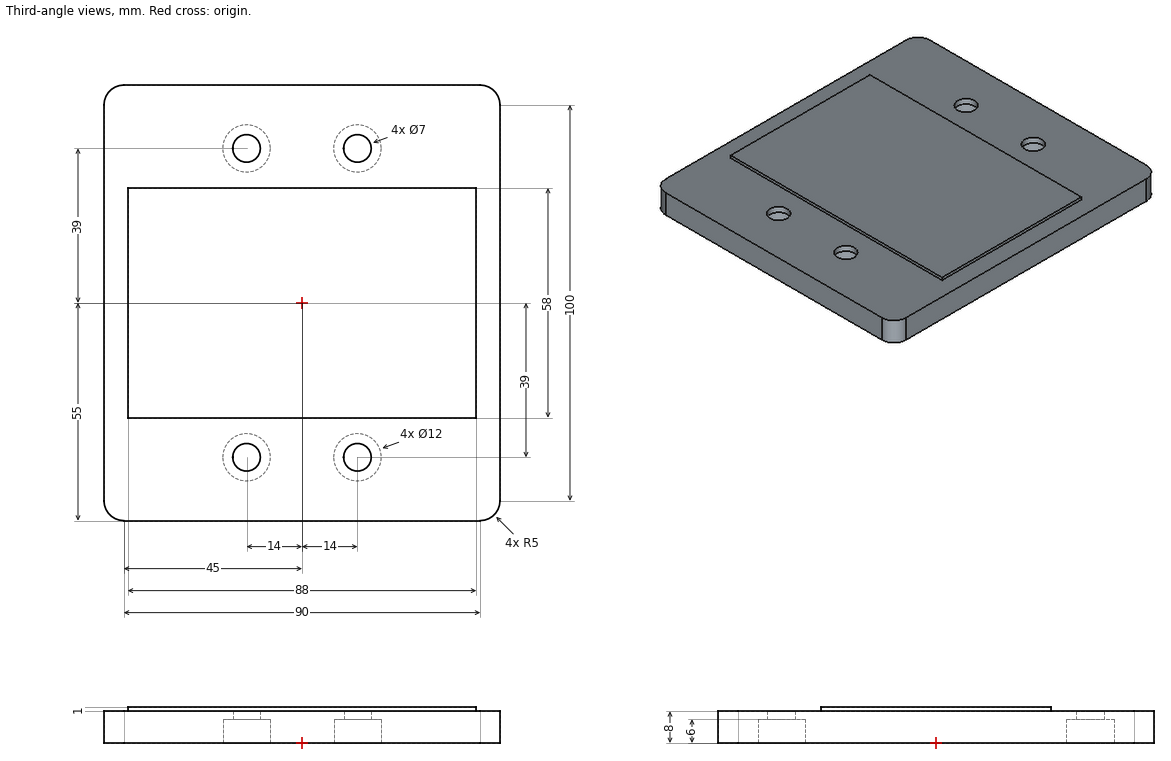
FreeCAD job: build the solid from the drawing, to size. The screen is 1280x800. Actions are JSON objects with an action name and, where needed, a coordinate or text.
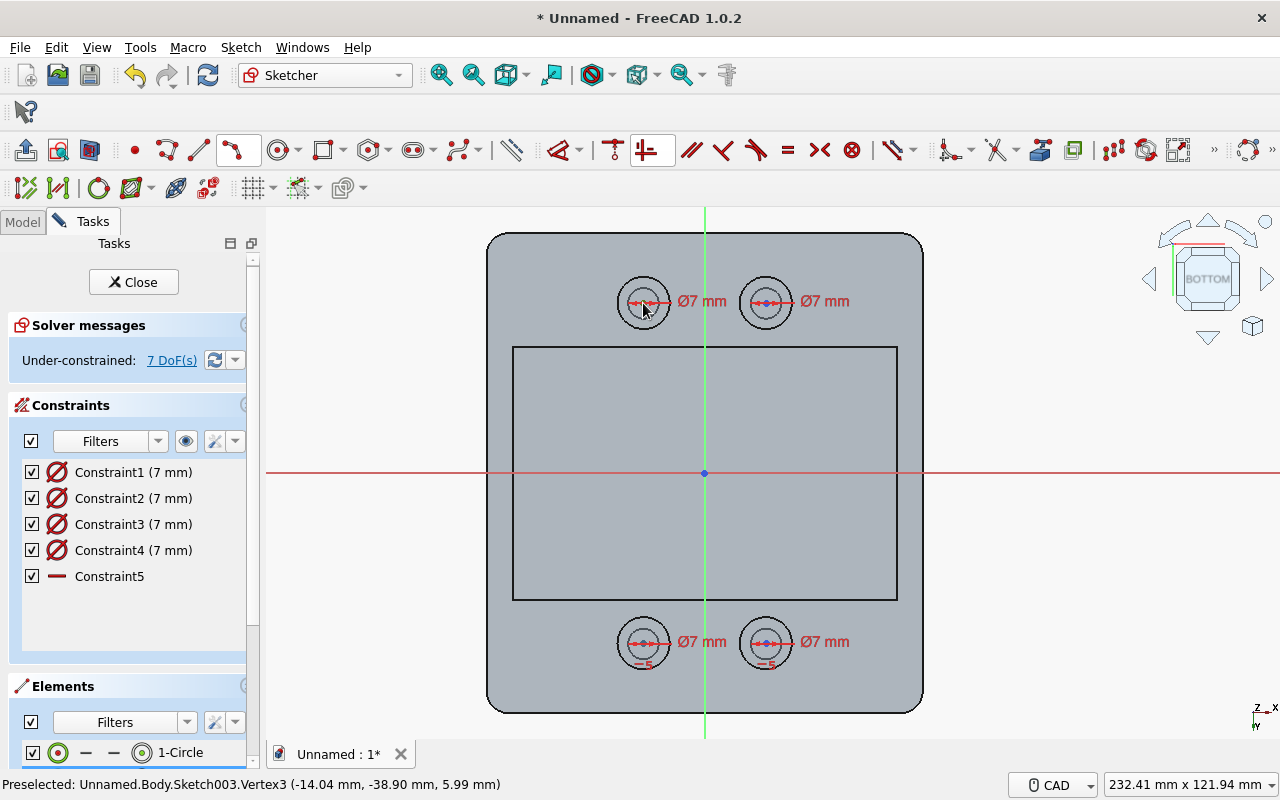
{"action": "key", "text": "v"}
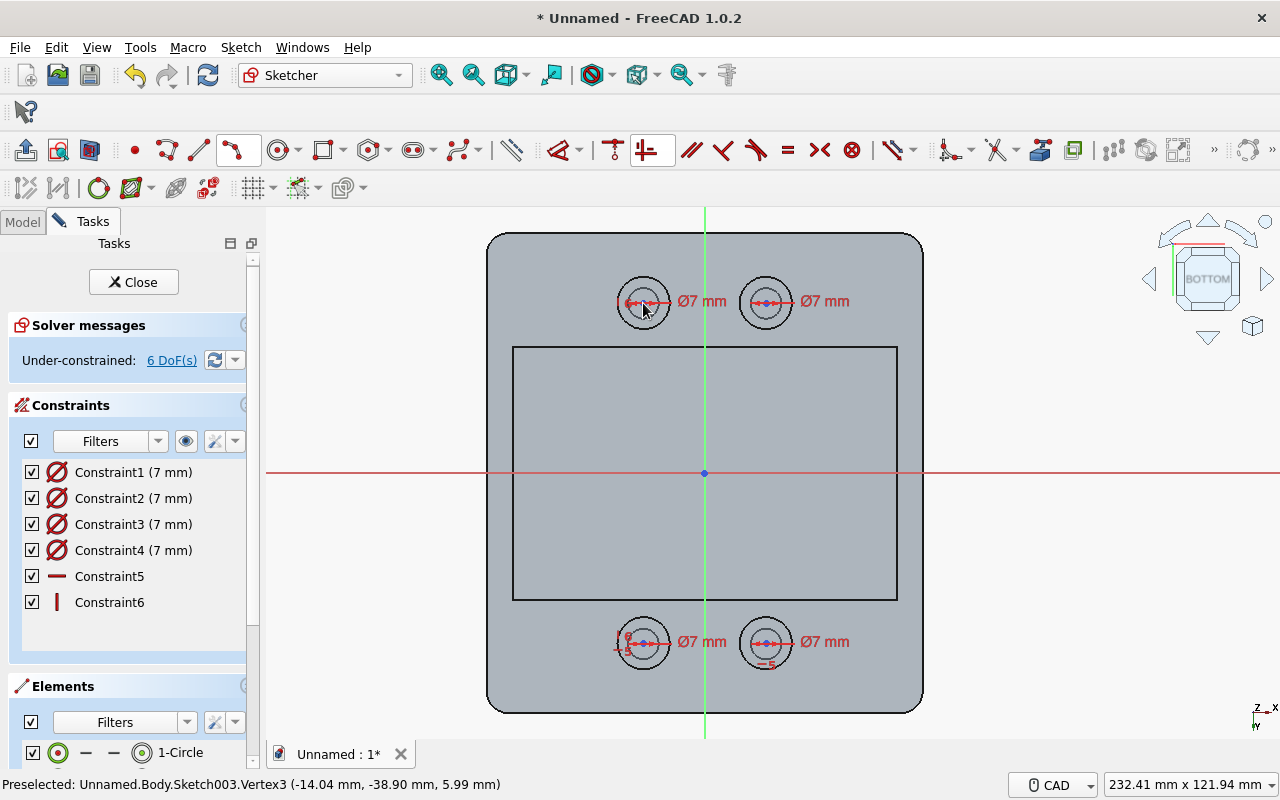
{"action": "left_click", "coordinate": [766, 644]}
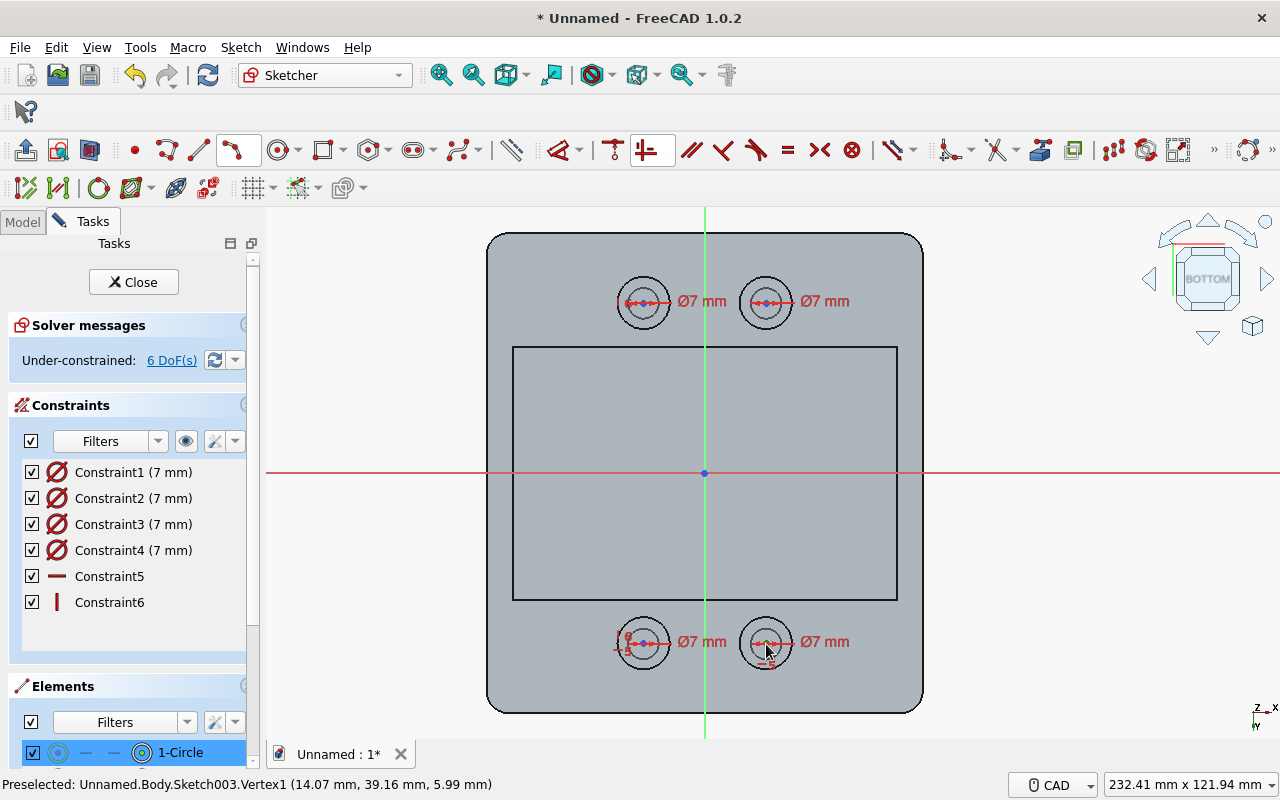
{"action": "left_click", "coordinate": [766, 303]}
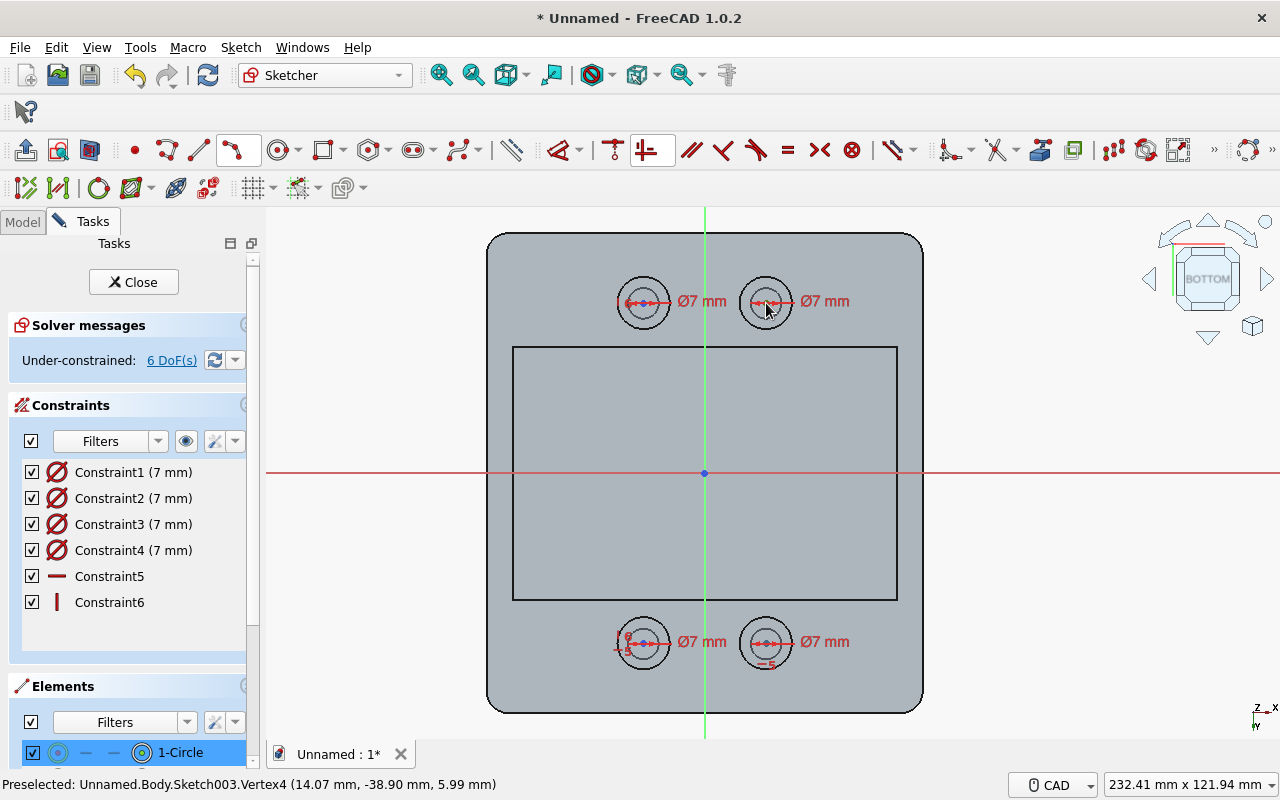
{"action": "key", "text": "v"}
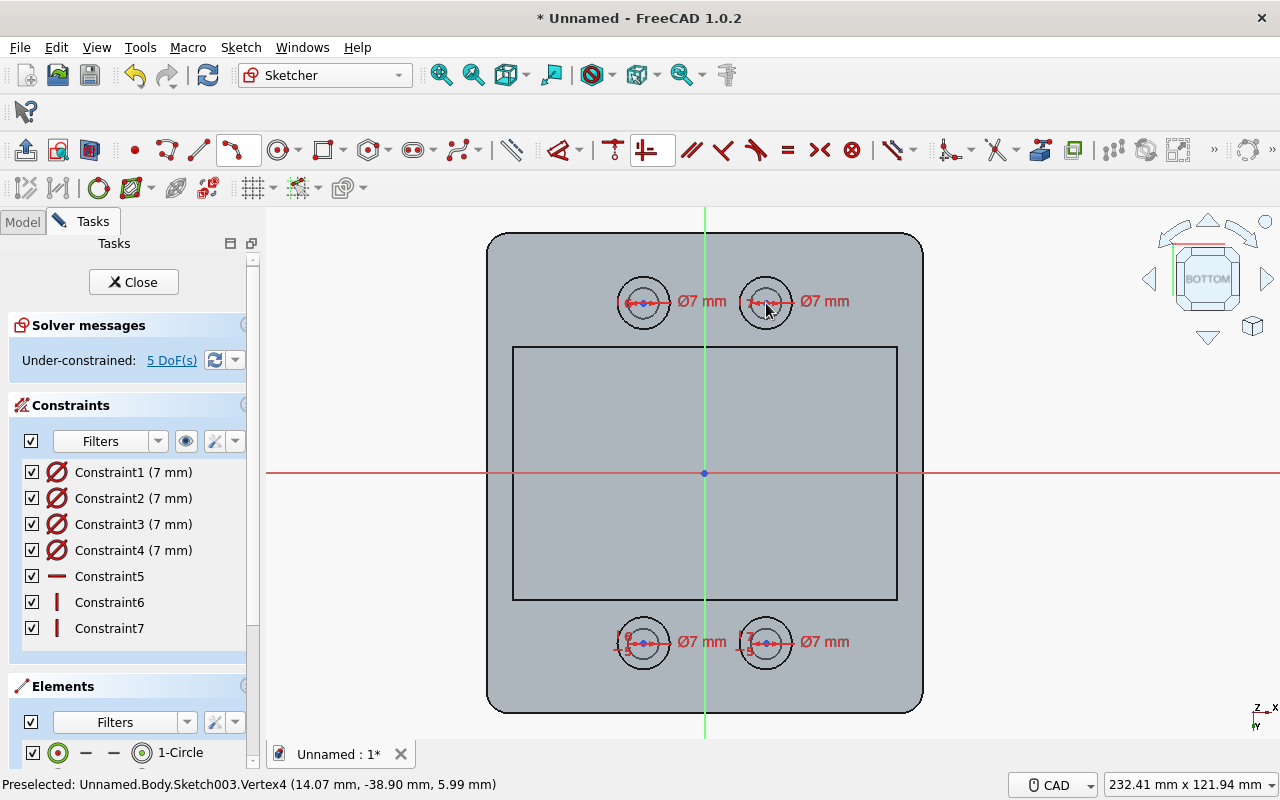
{"action": "left_click", "coordinate": [643, 303]}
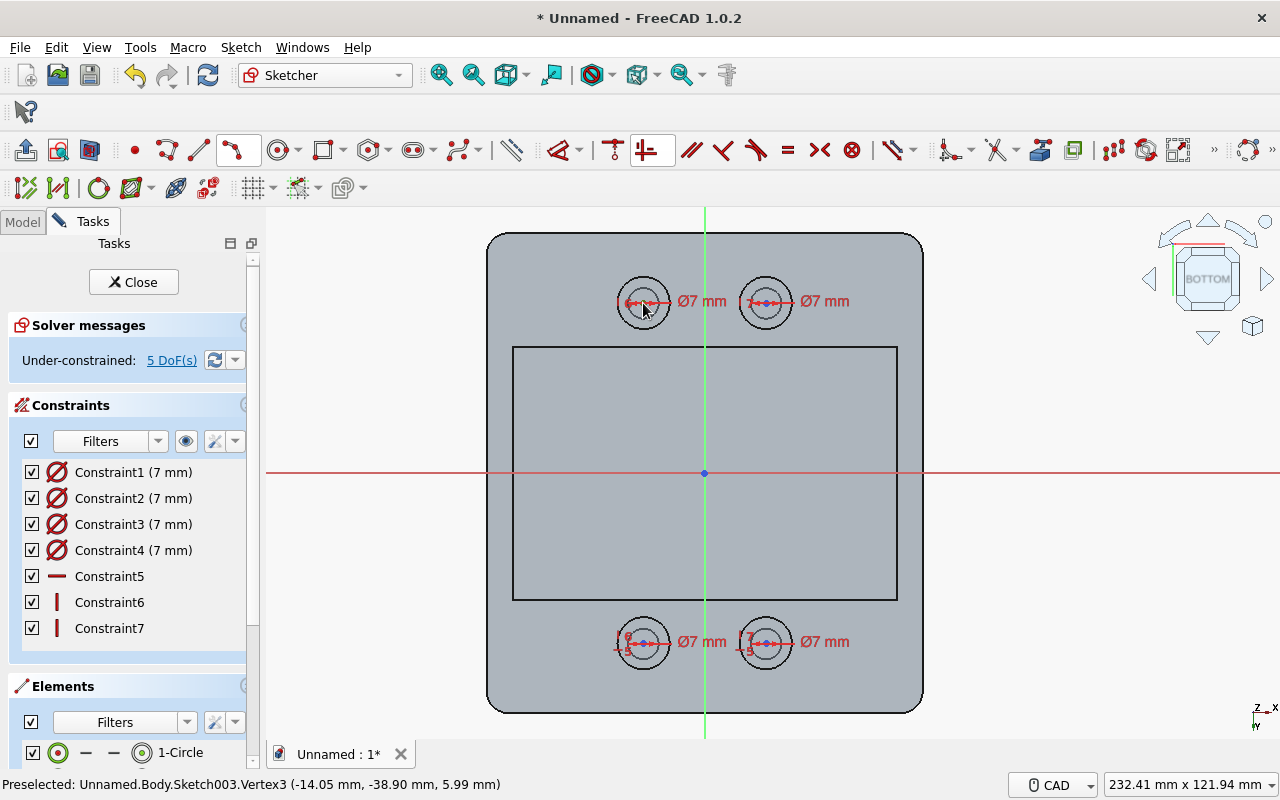
{"action": "left_click", "coordinate": [766, 303]}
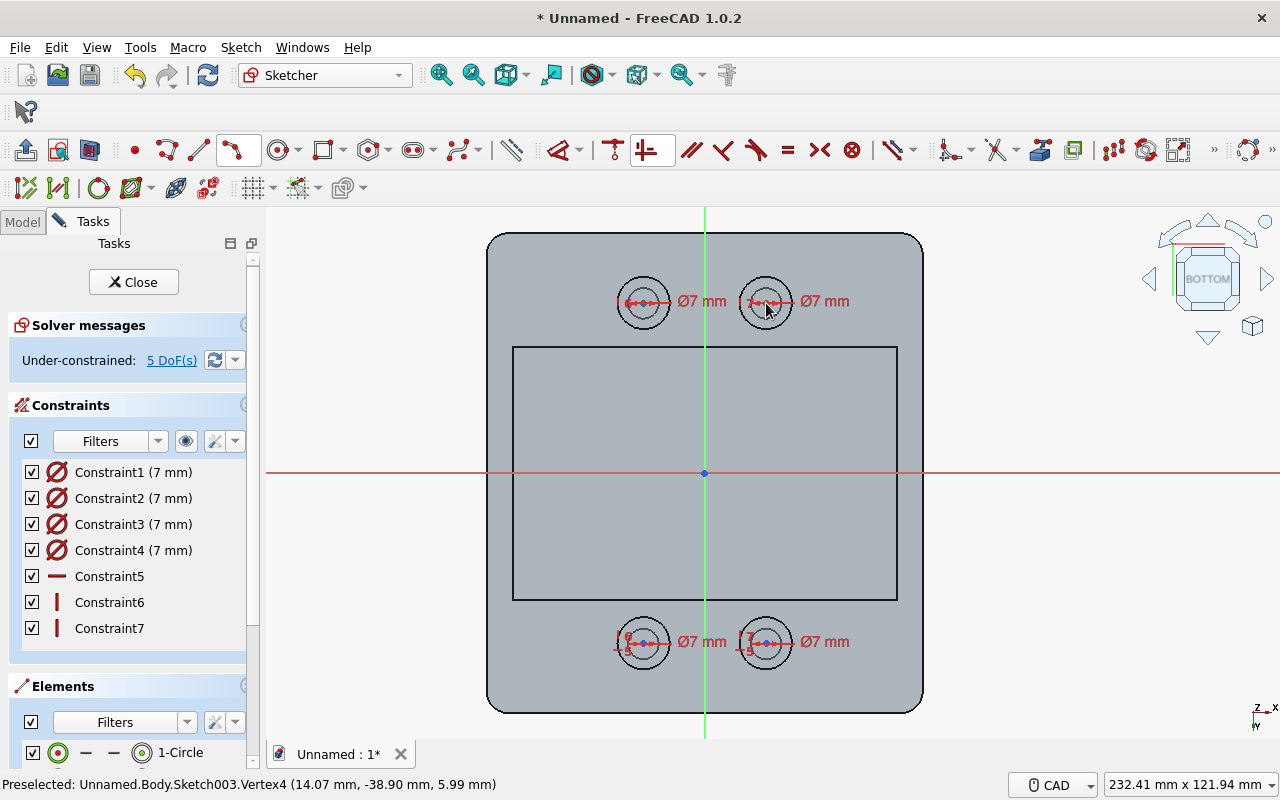
{"action": "key", "text": "h"}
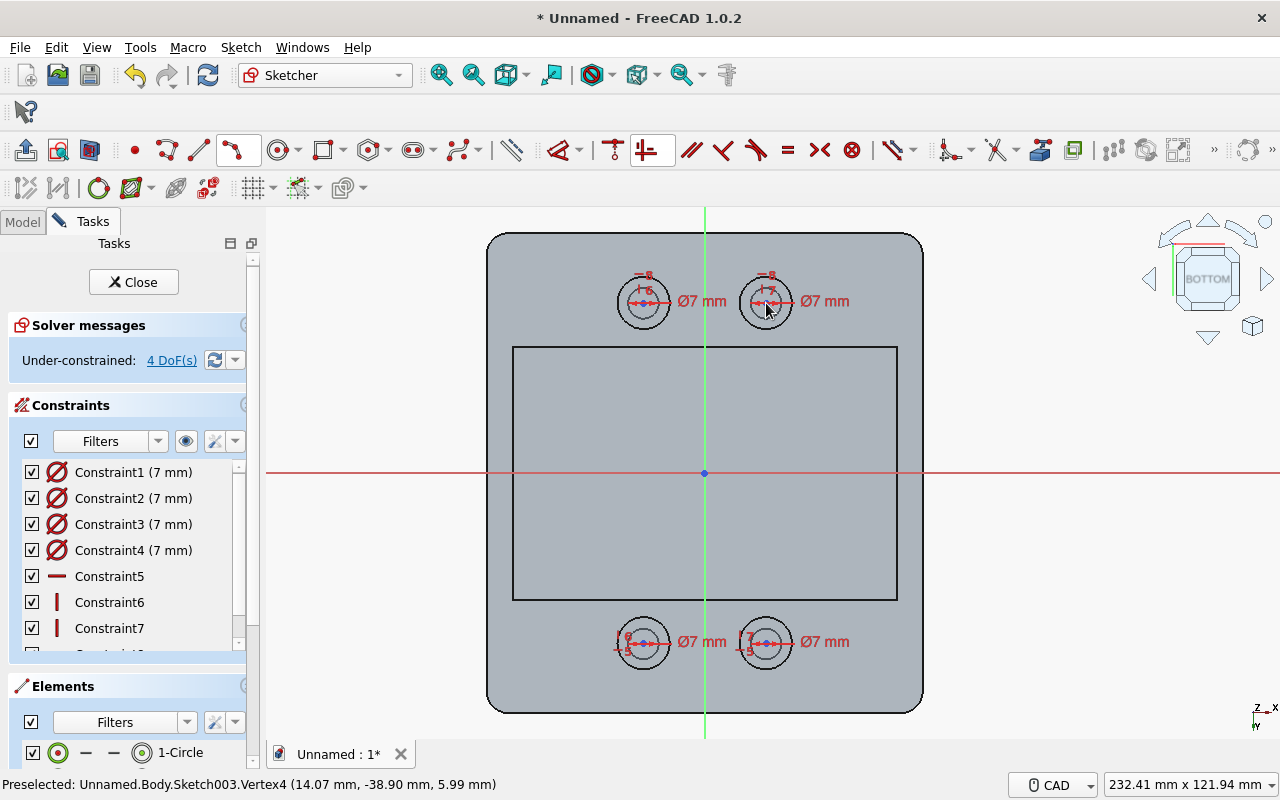
{"action": "left_click", "coordinate": [558, 150]}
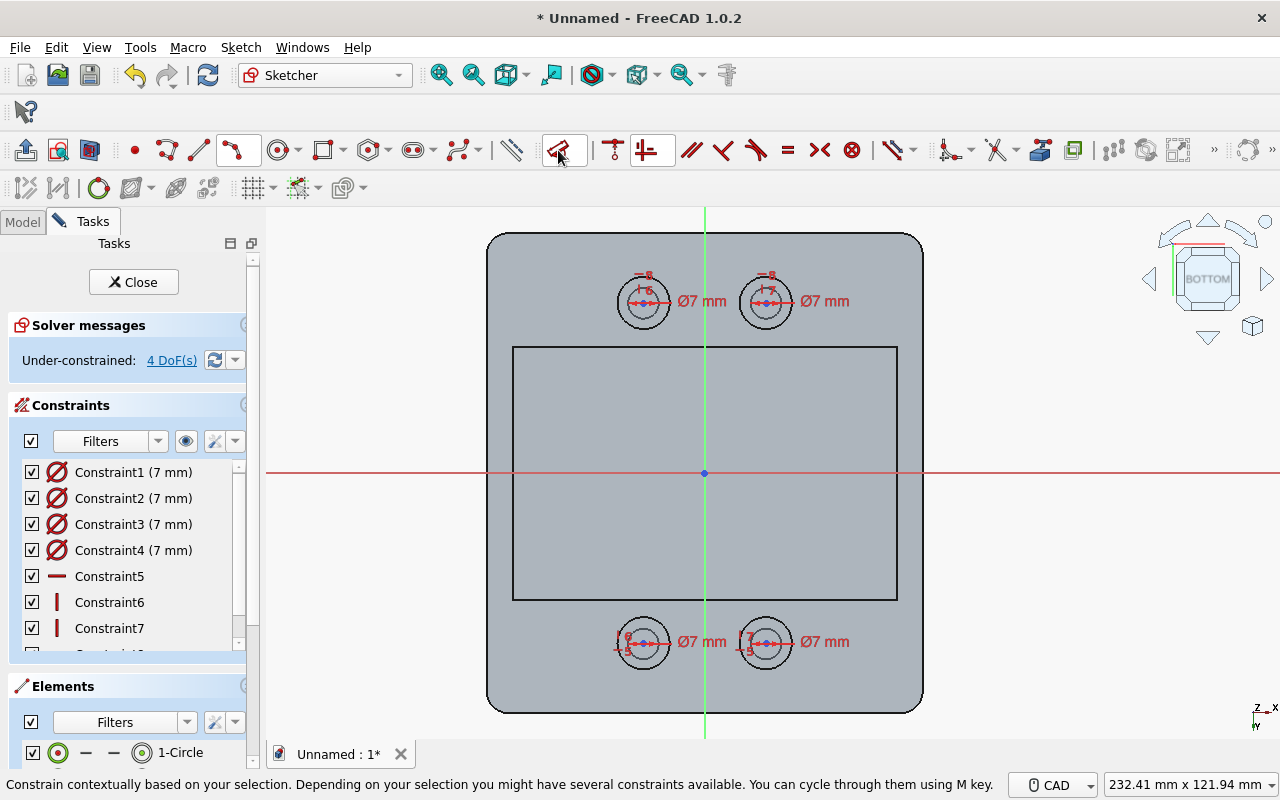
{"action": "left_click", "coordinate": [766, 644]}
{"action": "left_click", "coordinate": [735, 678]}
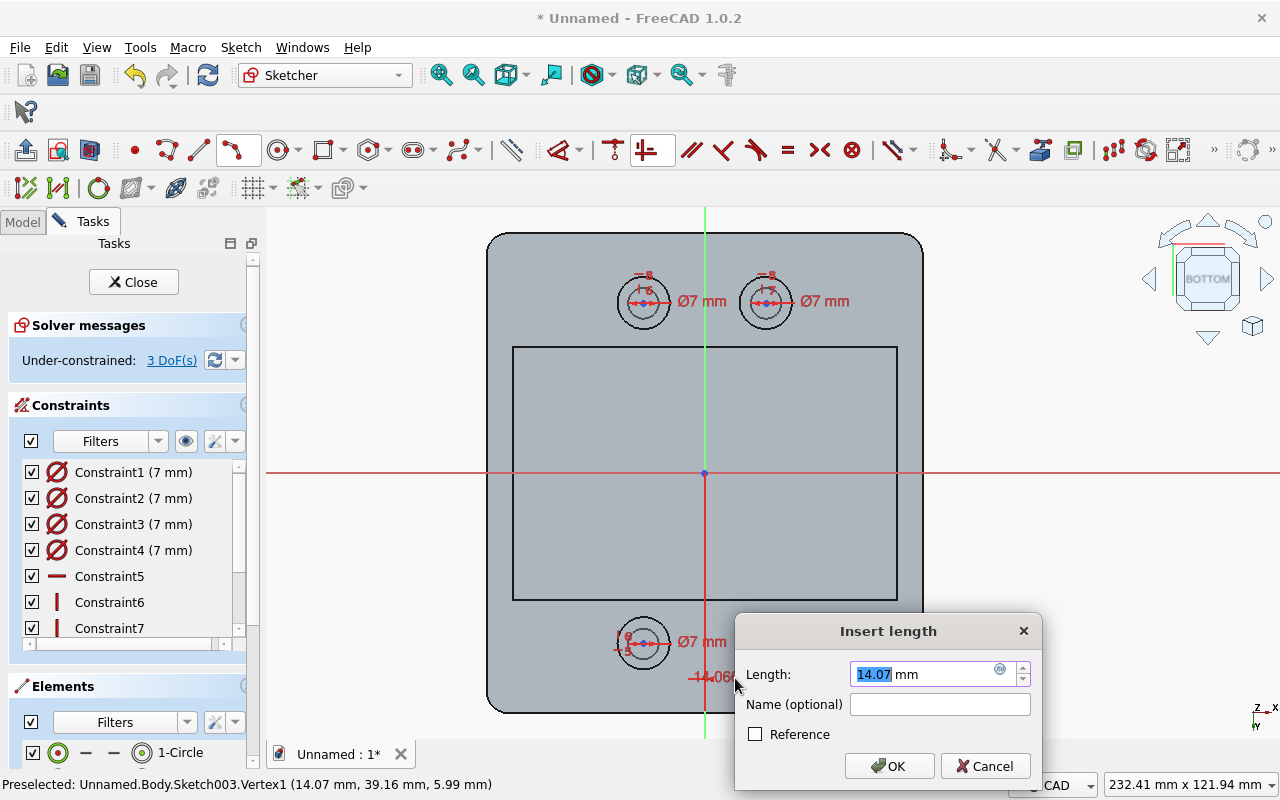
{"action": "type", "text": "14"}
{"action": "key", "text": "Return"}